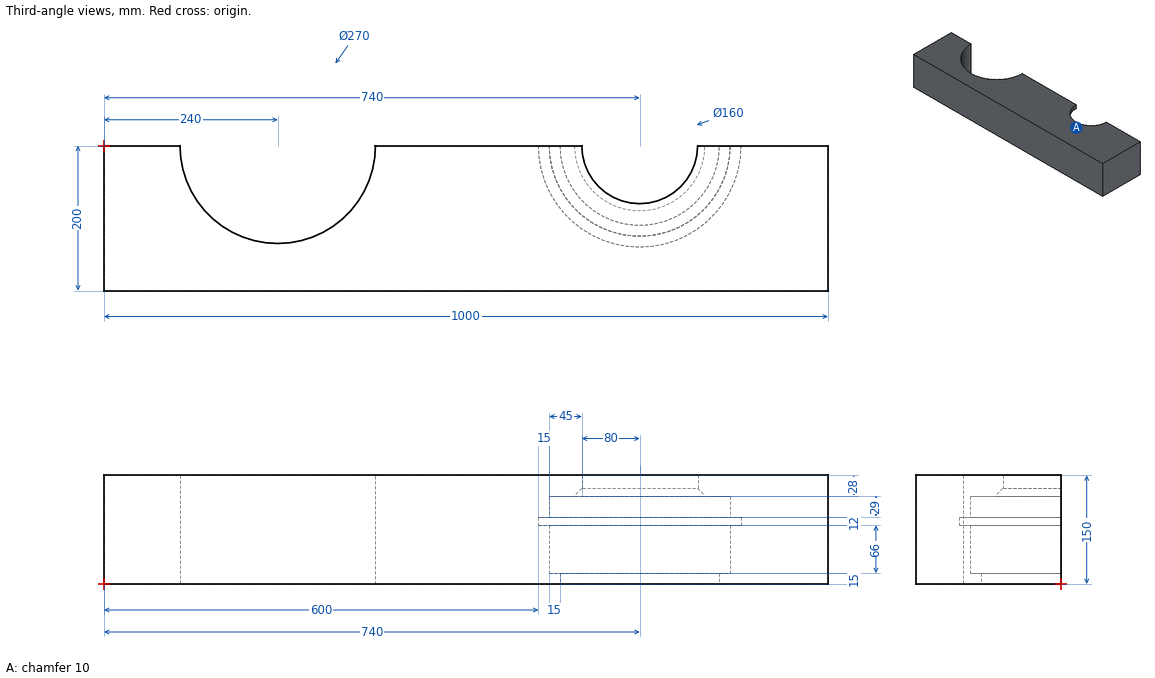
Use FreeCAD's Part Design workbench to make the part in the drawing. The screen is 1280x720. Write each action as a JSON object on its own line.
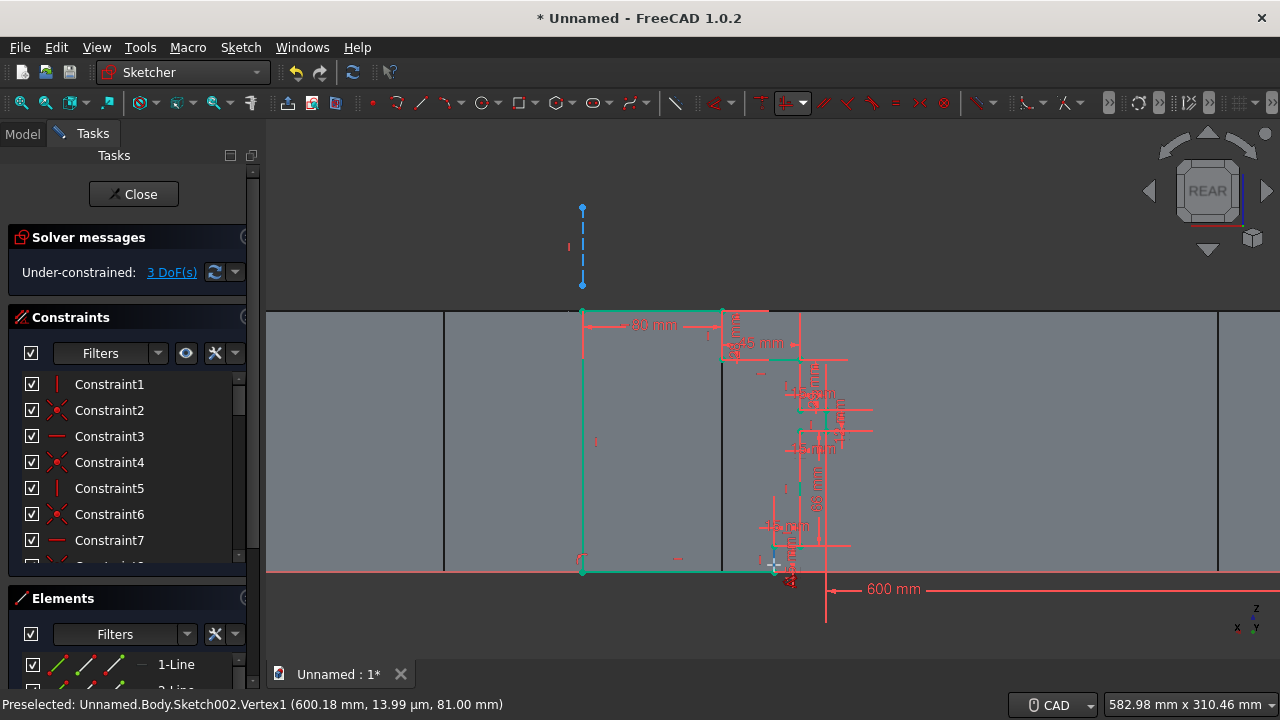
{"action": "left_click", "coordinate": [583, 285]}
{"action": "left_click", "coordinate": [727, 606]}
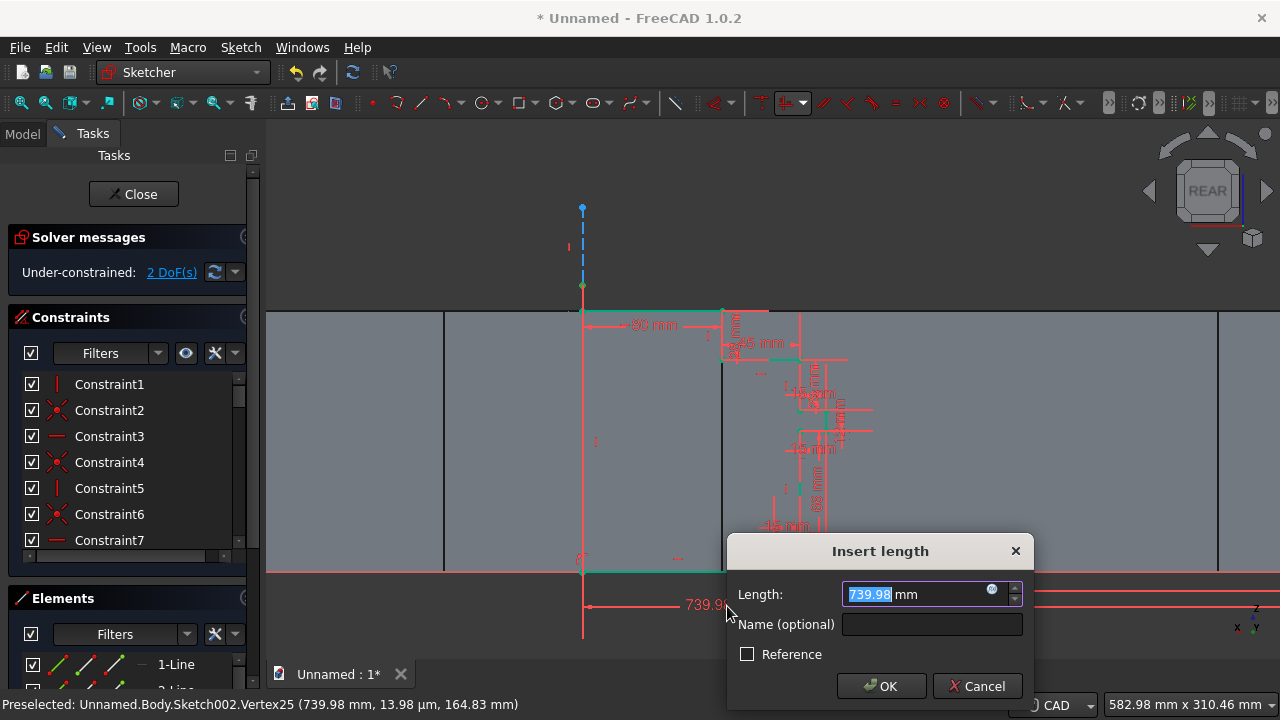
{"action": "type", "text": "740"}
{"action": "key", "text": "Return"}
{"action": "key", "text": "Escape"}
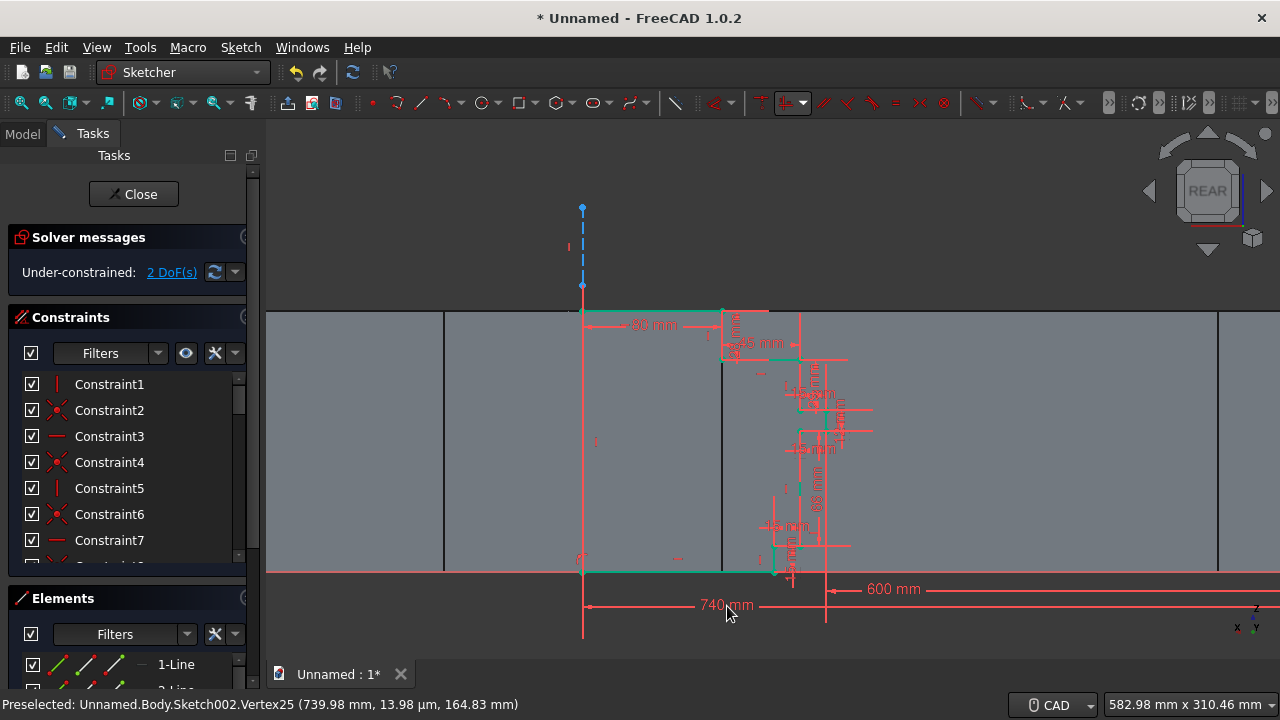
{"action": "left_click", "coordinate": [134, 194]}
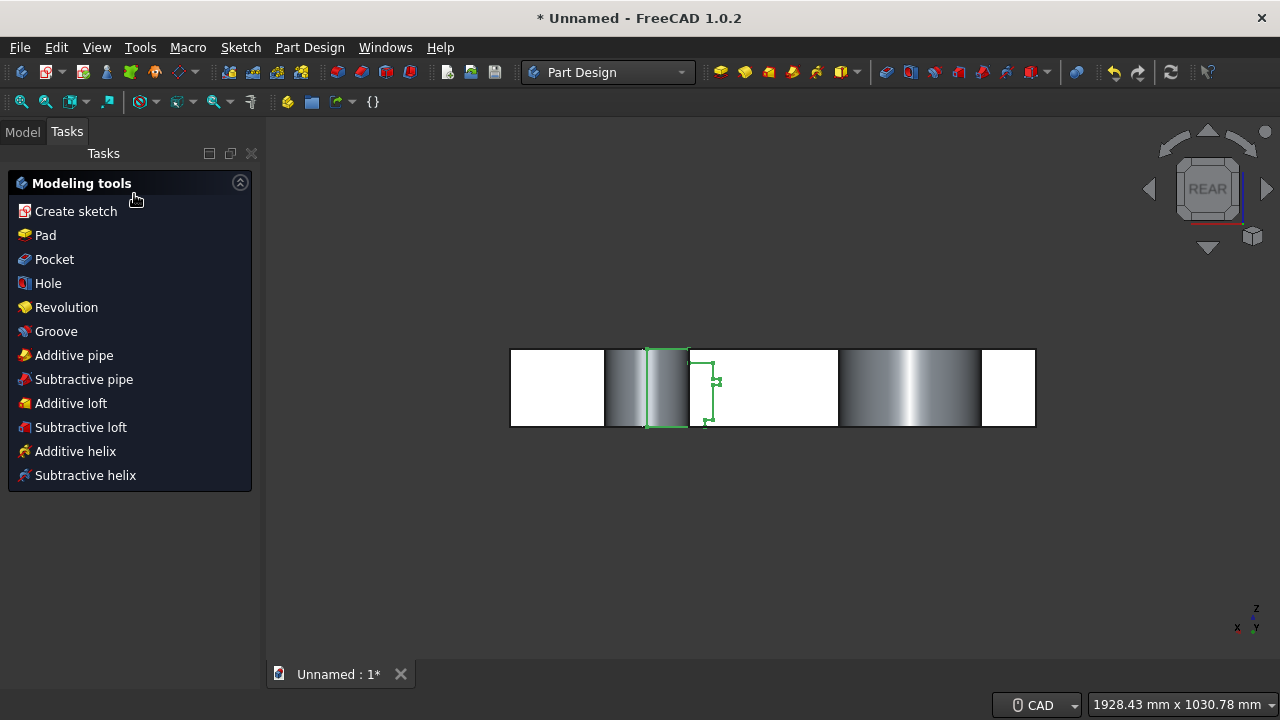
{"action": "left_click", "coordinate": [936, 72]}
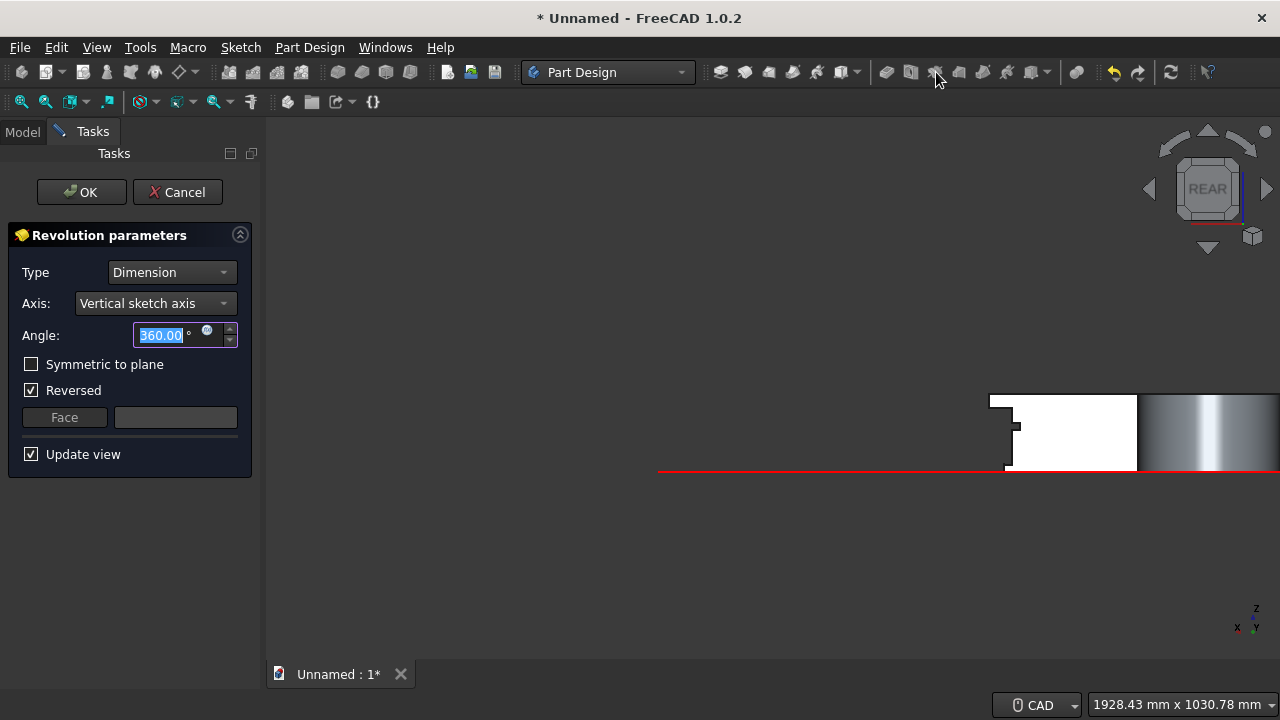
{"action": "left_click", "coordinate": [156, 304]}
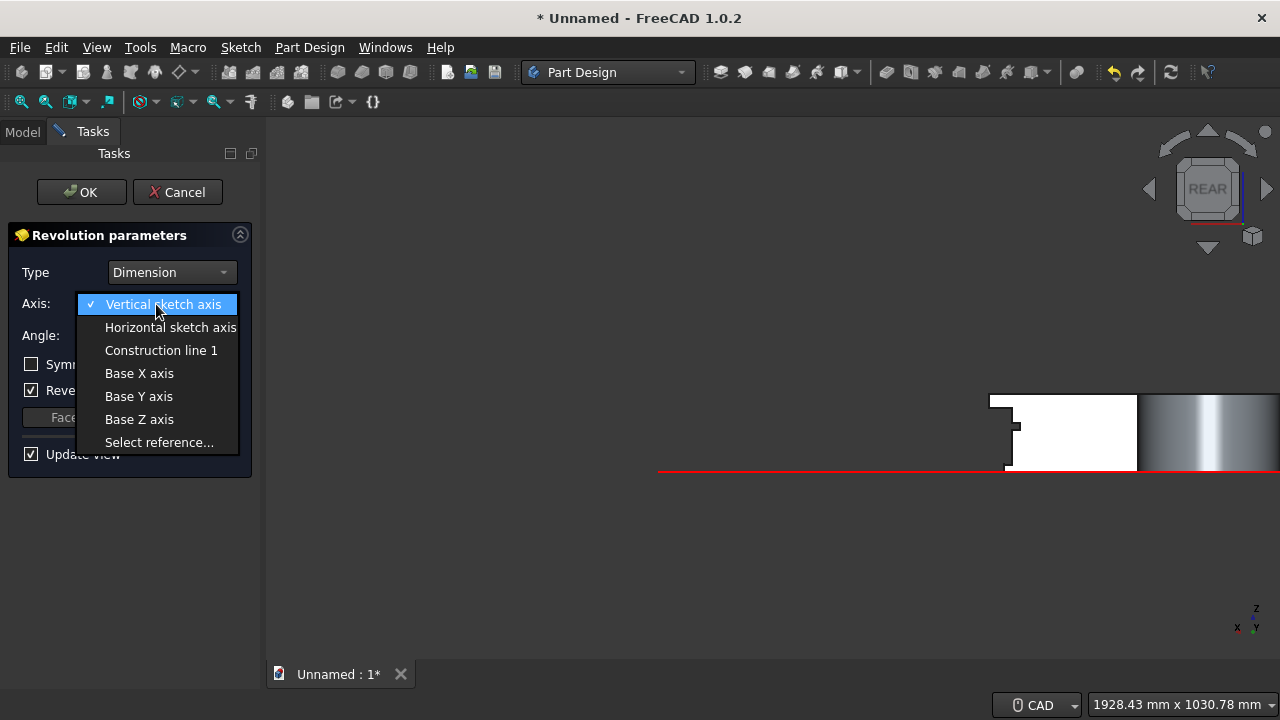
{"action": "left_click", "coordinate": [156, 350]}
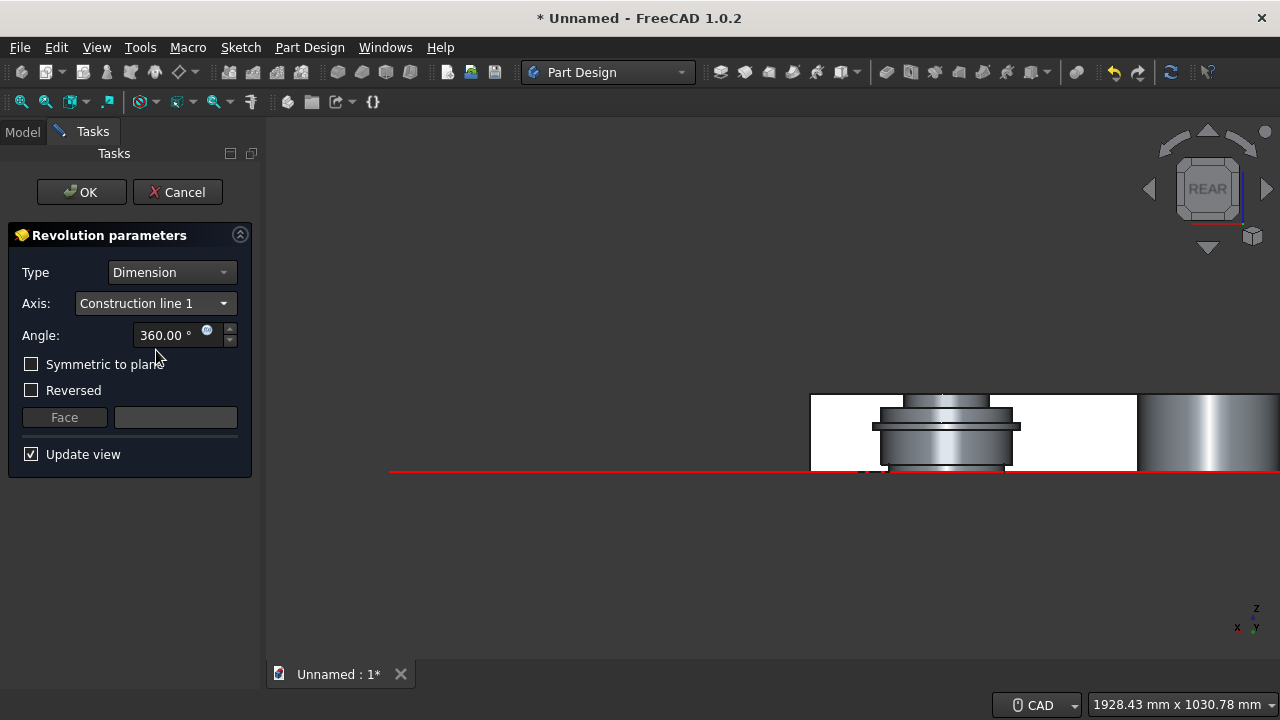
{"action": "left_click", "coordinate": [82, 192]}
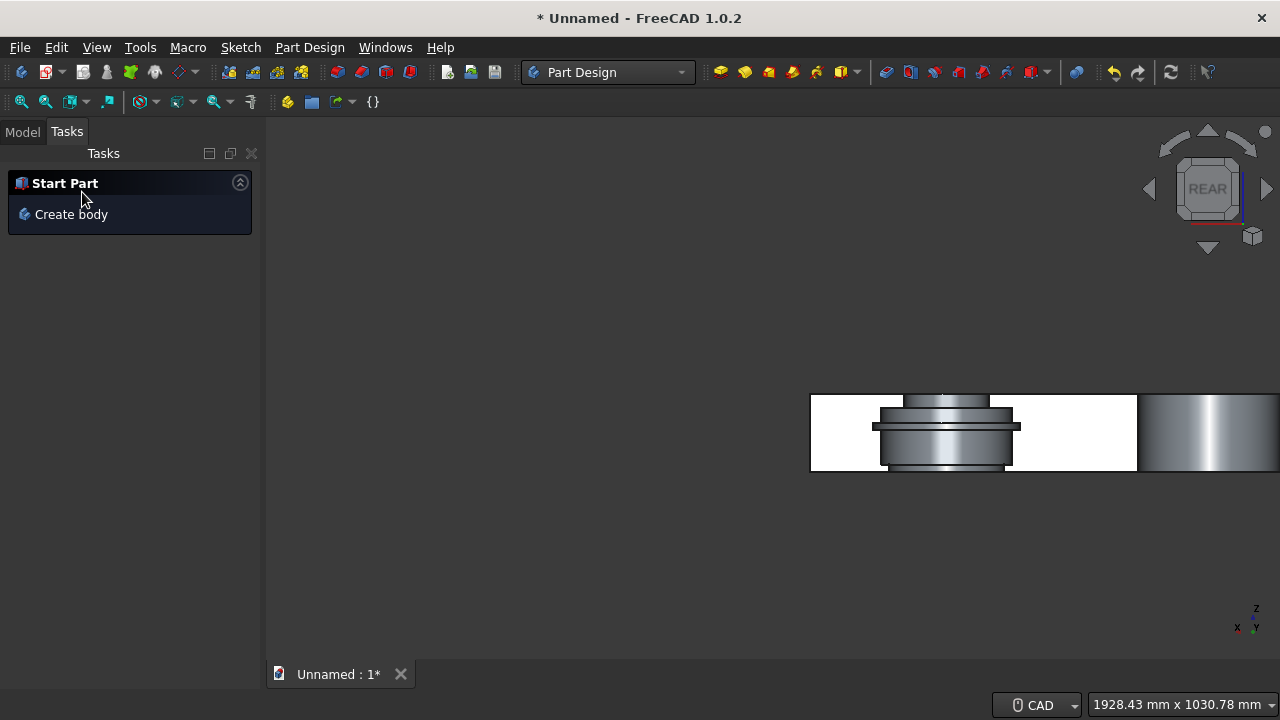
{"action": "left_click", "coordinate": [22, 102]}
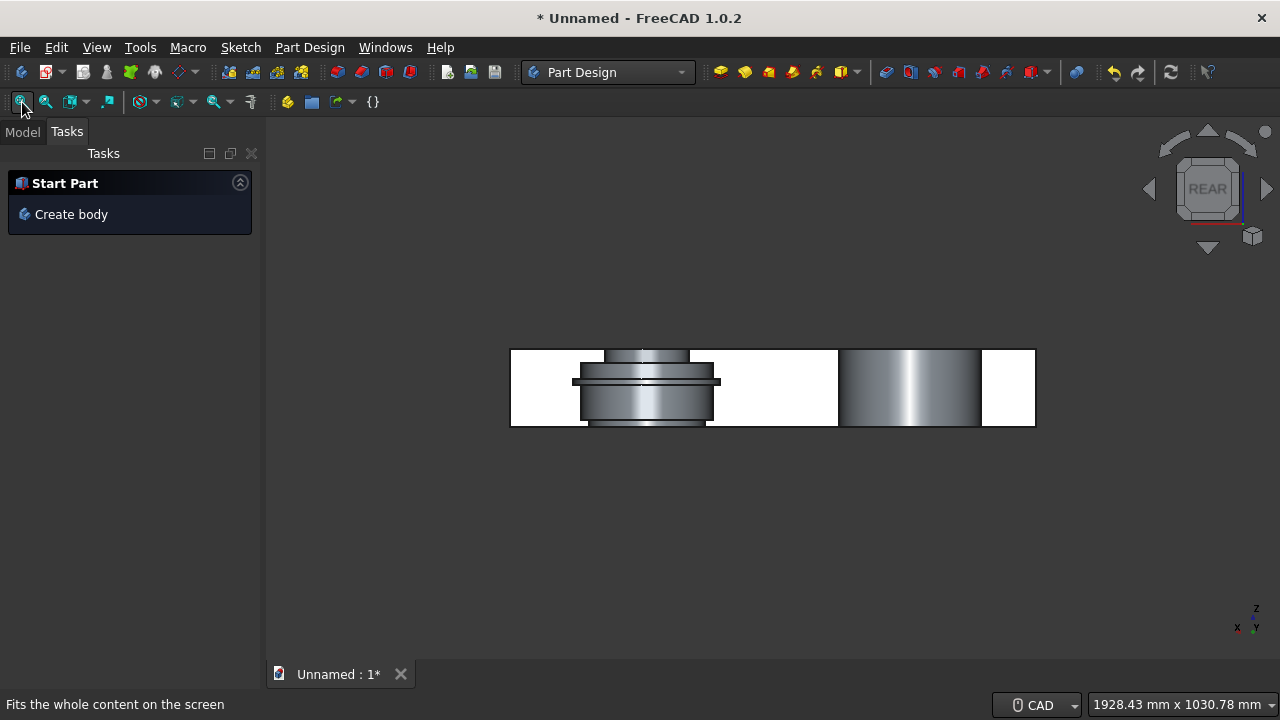
{"action": "key", "text": "0"}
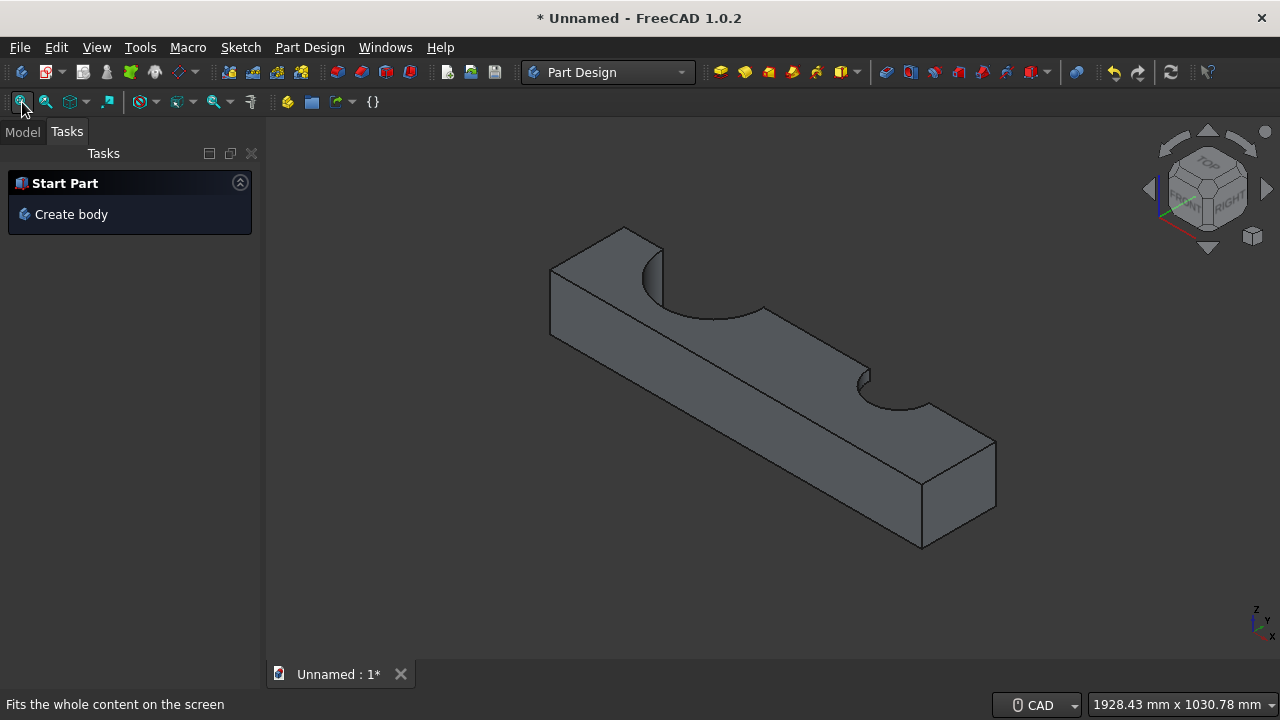
{"action": "key", "text": "2"}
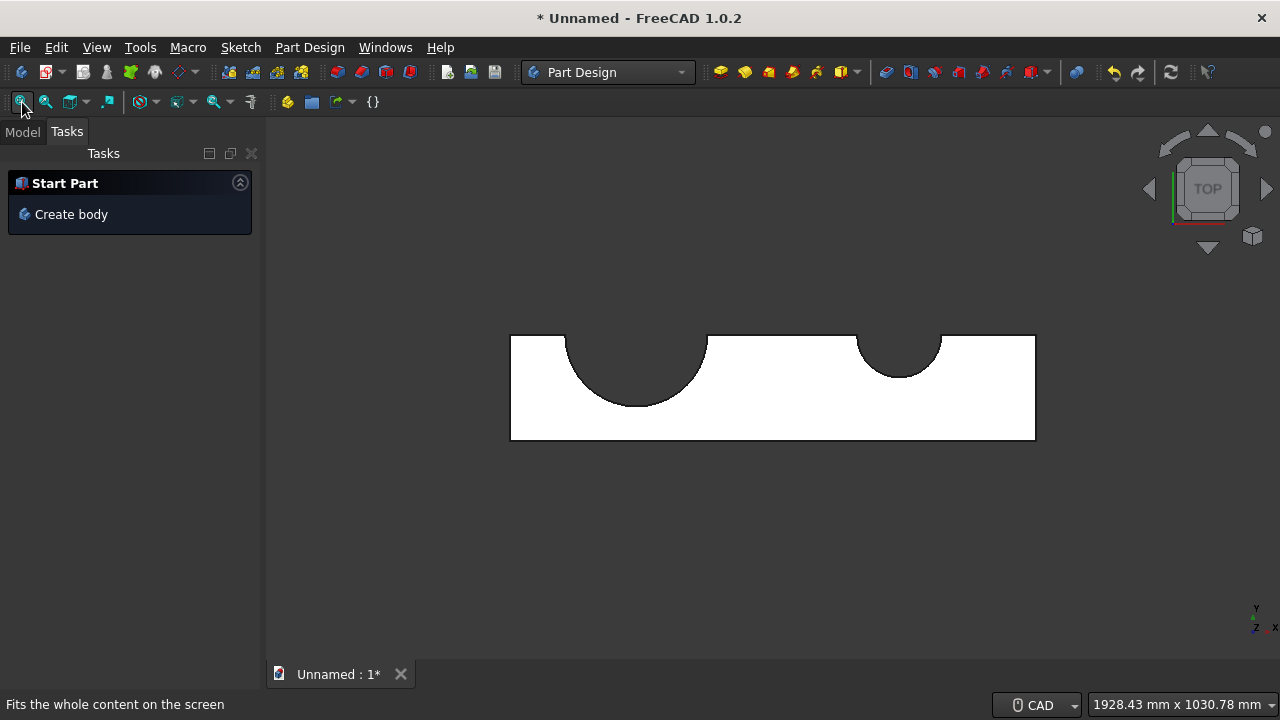
{"action": "key", "text": "1"}